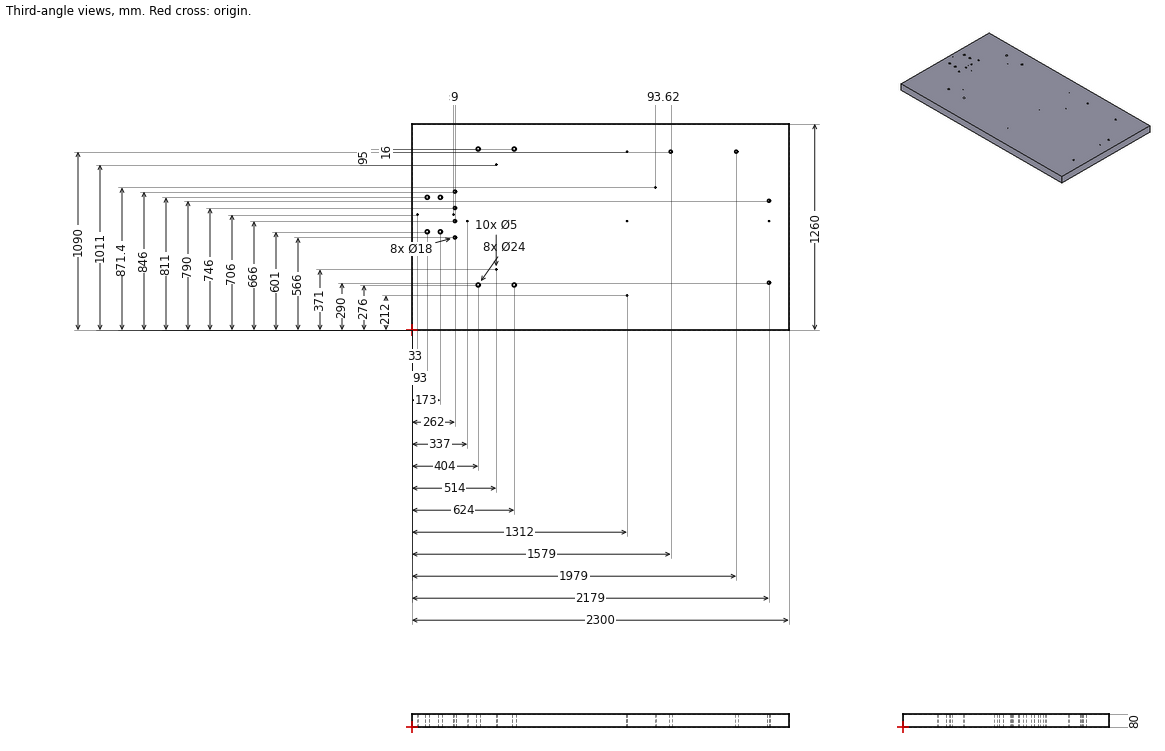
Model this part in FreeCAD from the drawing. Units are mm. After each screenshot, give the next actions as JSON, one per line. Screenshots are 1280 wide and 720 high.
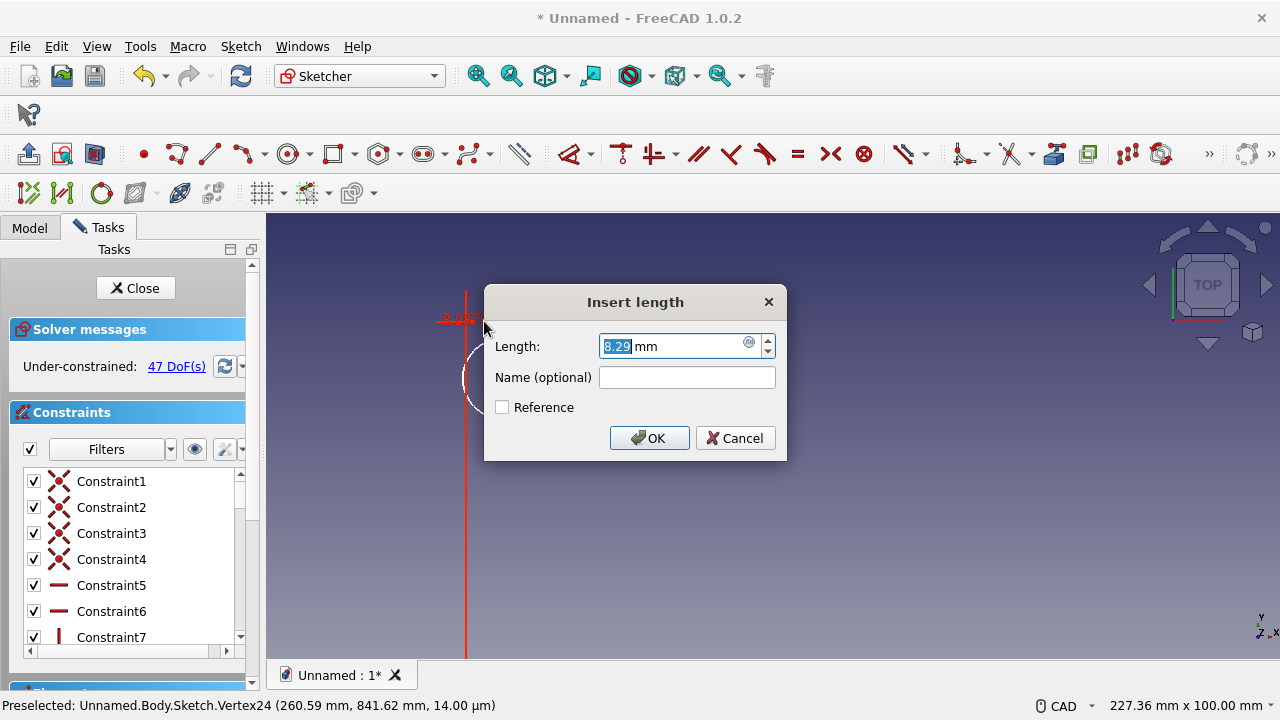
{"action": "type", "text": "9"}
{"action": "key", "text": "Return"}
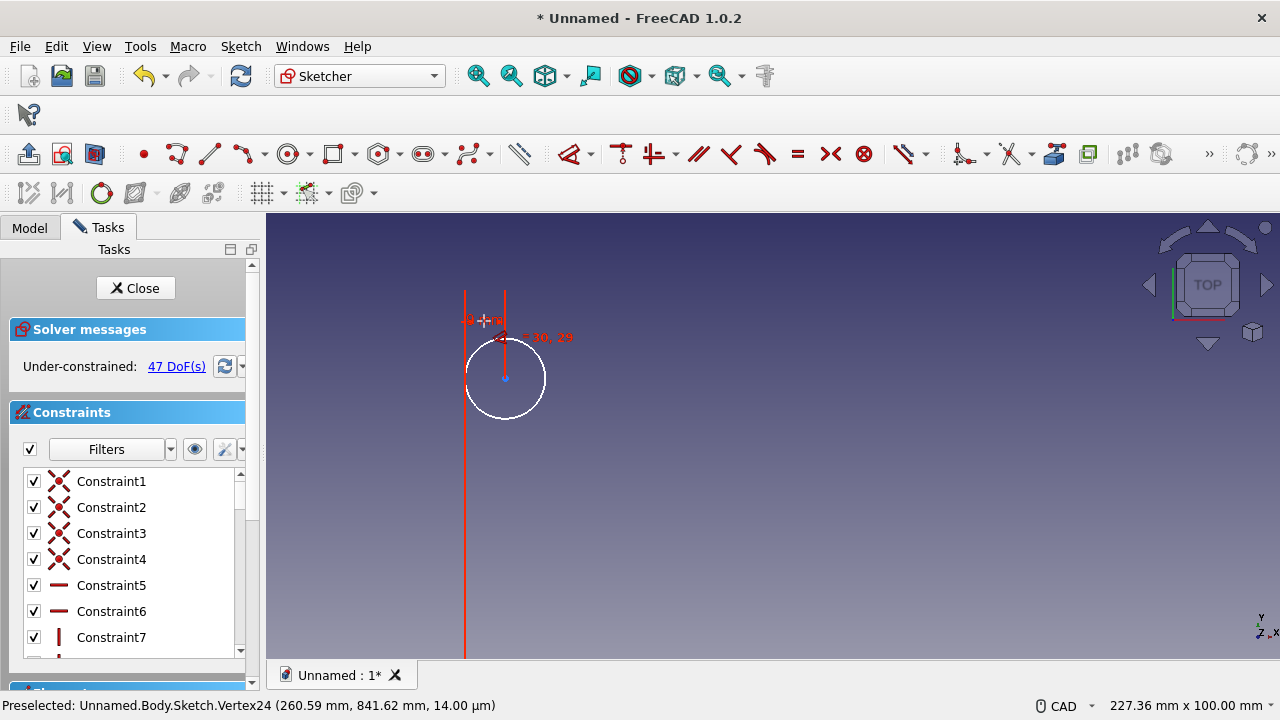
{"action": "scroll", "coordinate": [507, 390], "scroll_direction": "down", "scroll_amount": 15}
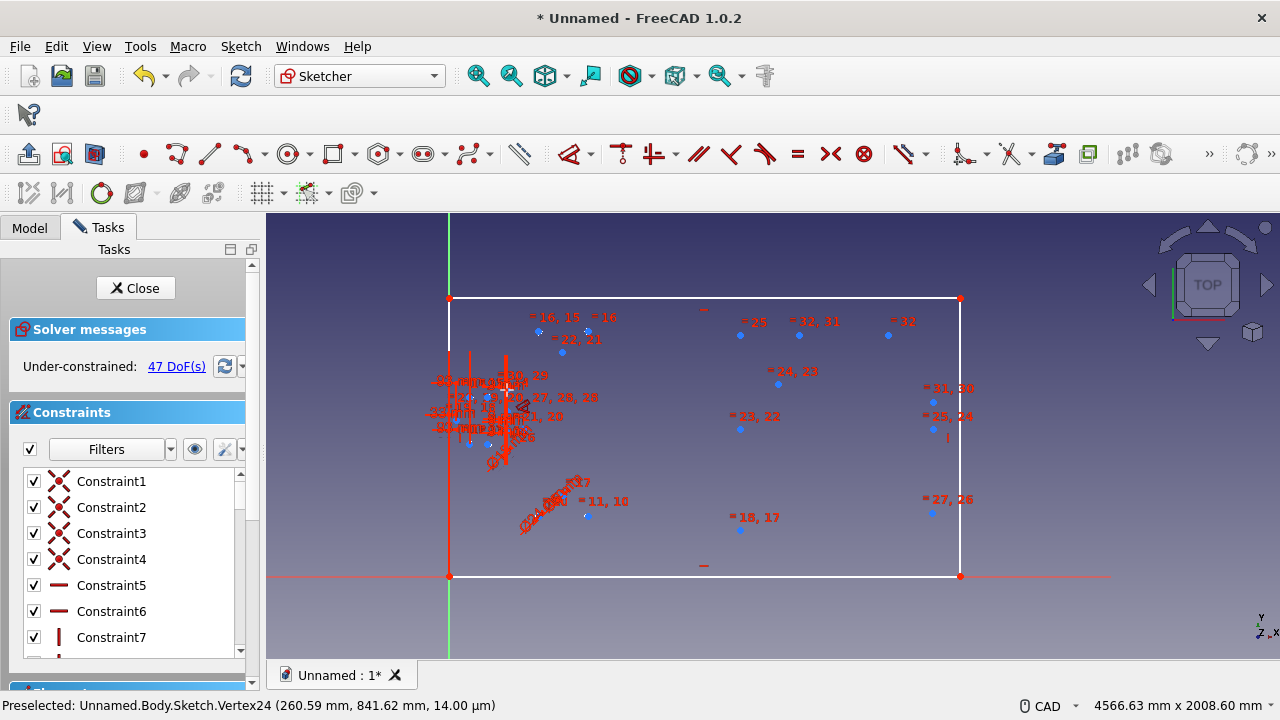
{"action": "left_click", "coordinate": [539, 516]}
{"action": "left_click", "coordinate": [494, 611]}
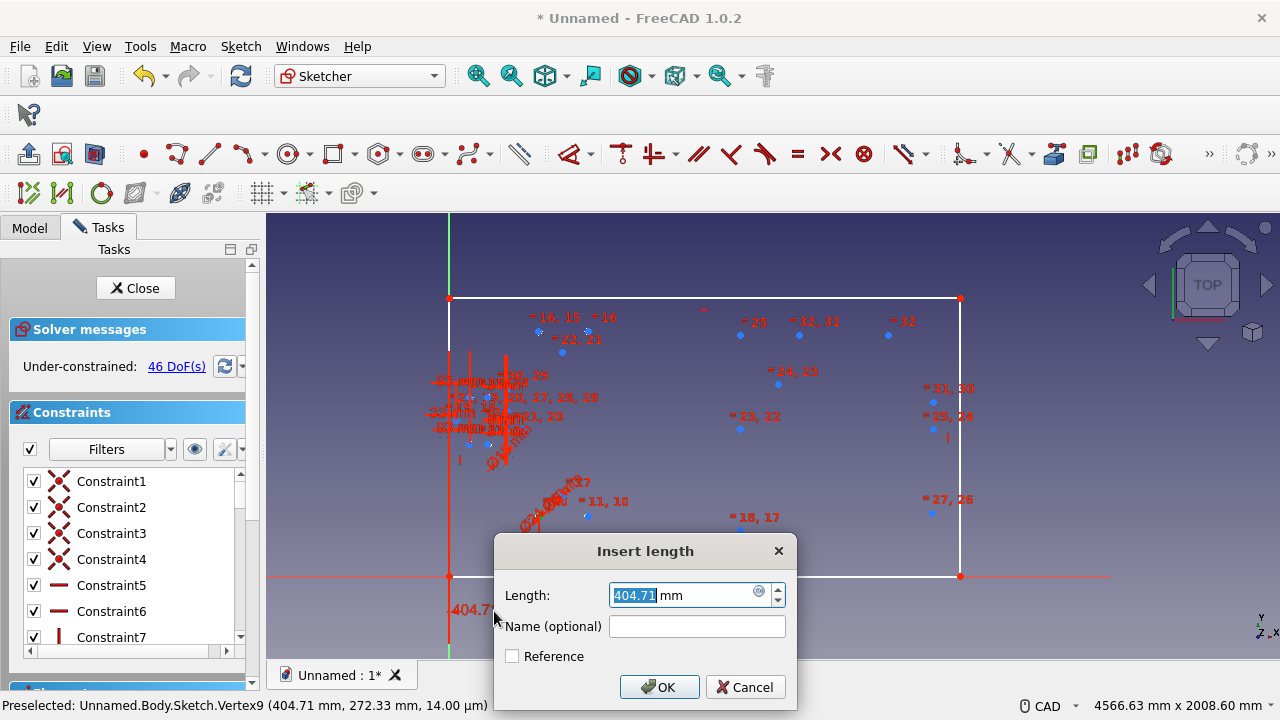
{"action": "type", "text": "404"}
{"action": "key", "text": "Return"}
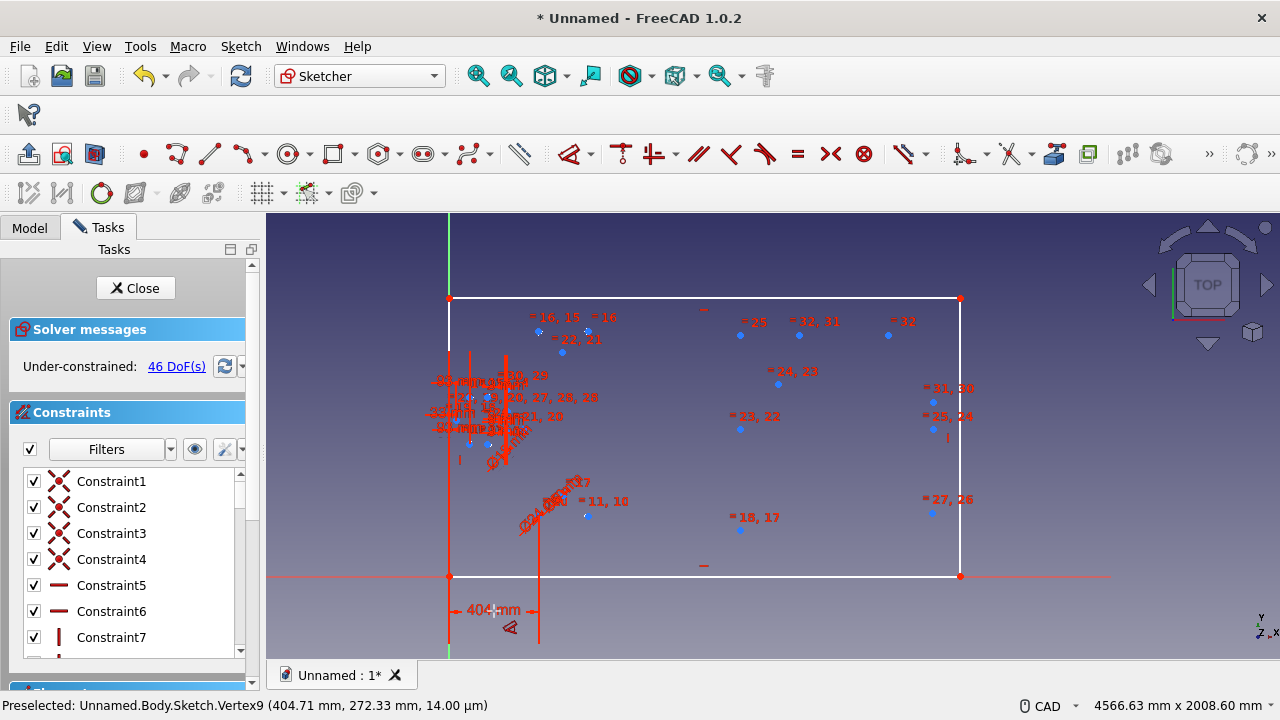
{"action": "left_click", "coordinate": [539, 516]}
{"action": "left_click", "coordinate": [415, 546]}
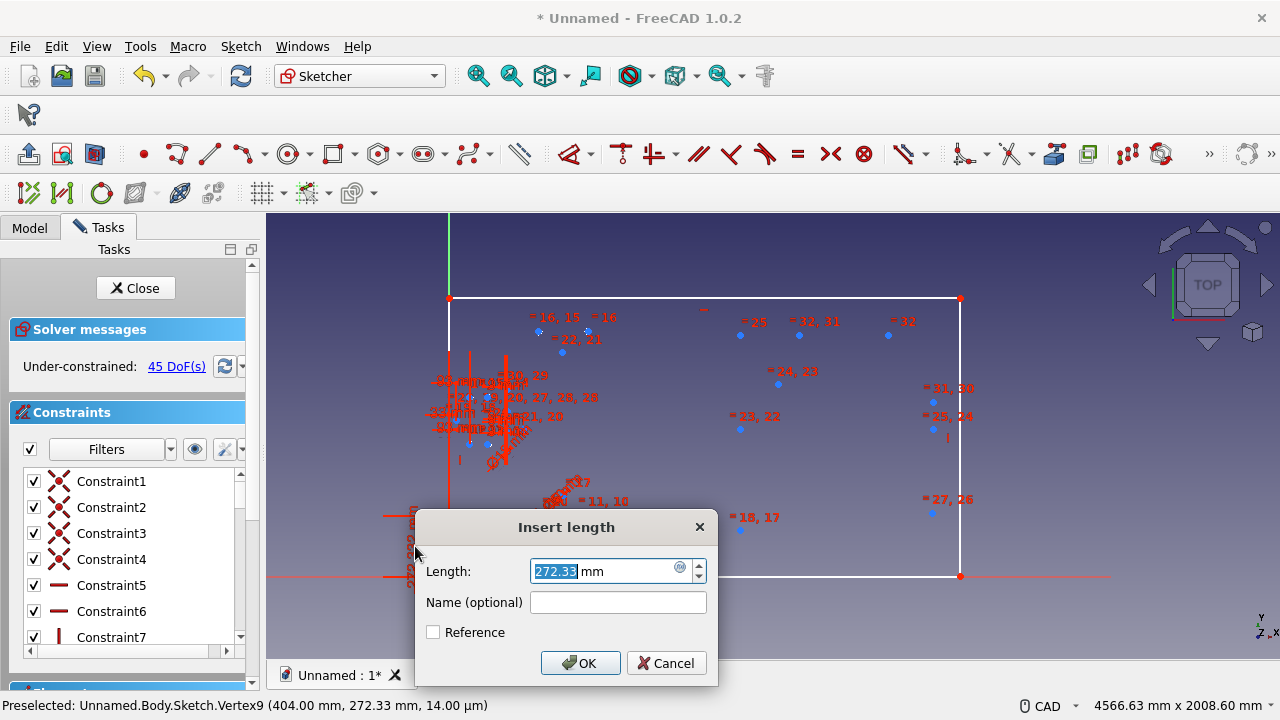
{"action": "type", "text": "276"}
{"action": "key", "text": "Return"}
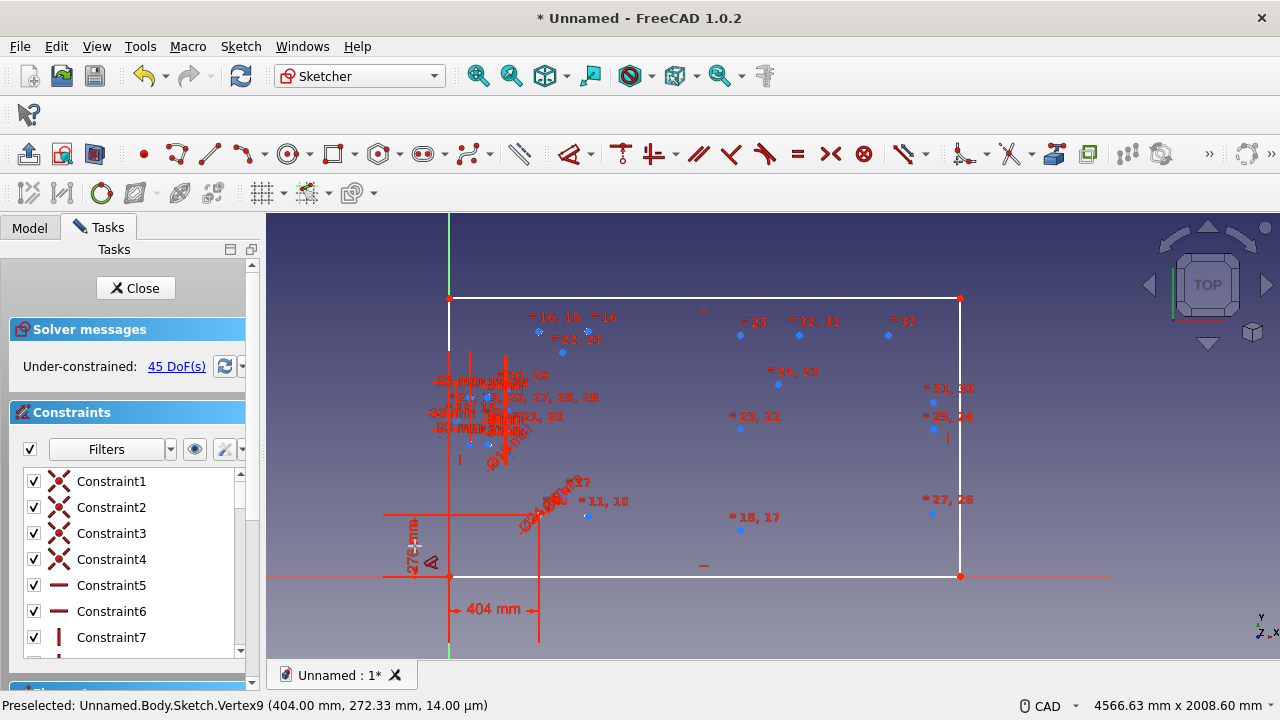
{"action": "left_click", "coordinate": [563, 495]}
{"action": "left_click", "coordinate": [532, 365]}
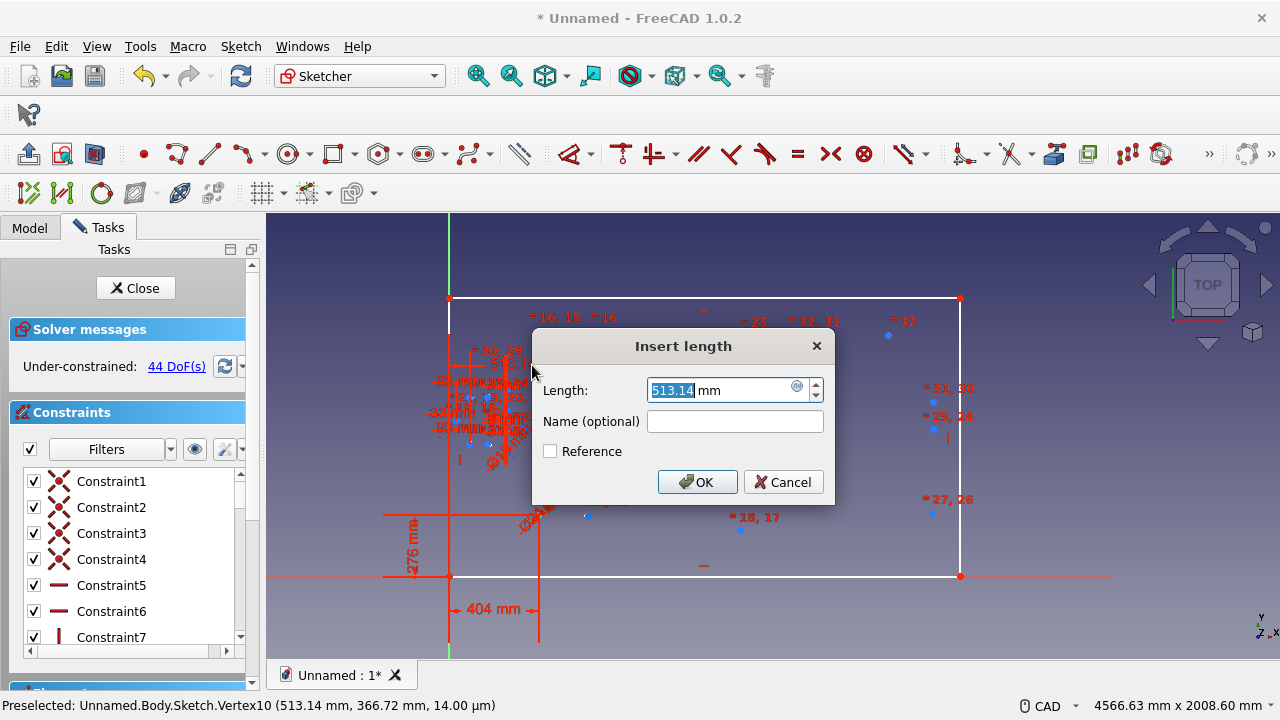
{"action": "type", "text": "514"}
{"action": "key", "text": "Return"}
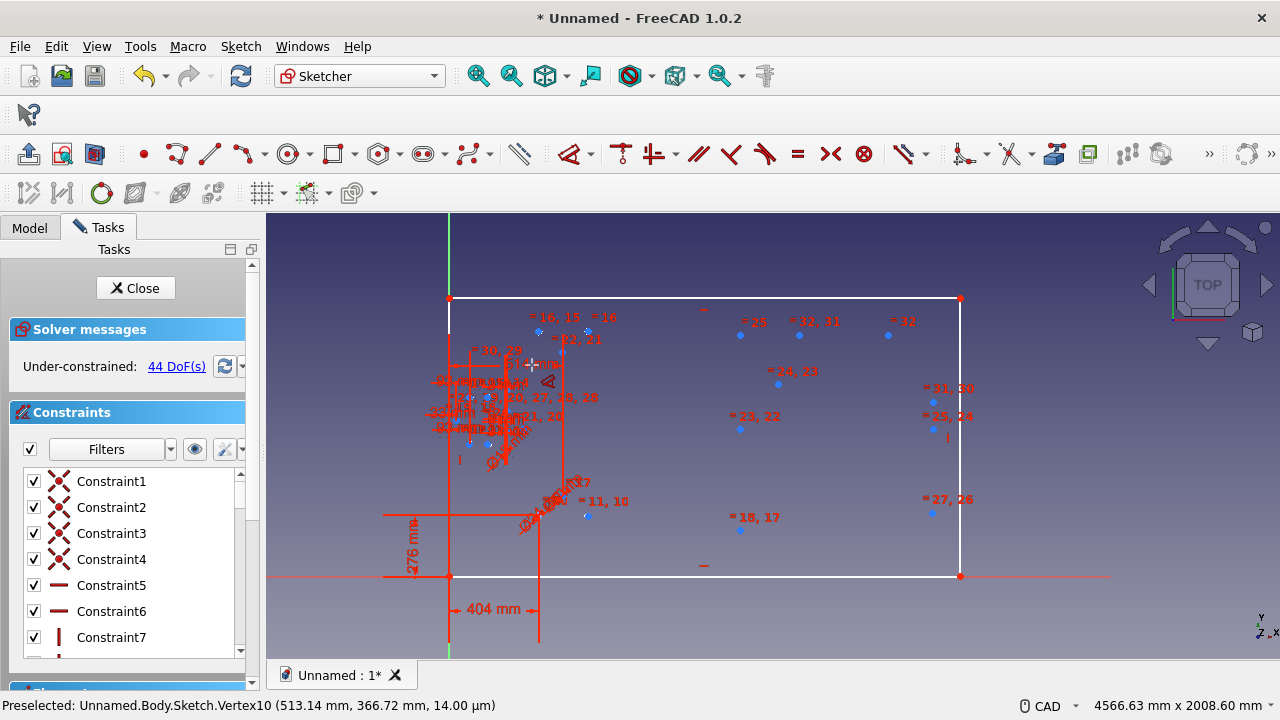
{"action": "left_click", "coordinate": [563, 495]}
{"action": "left_click", "coordinate": [415, 517]}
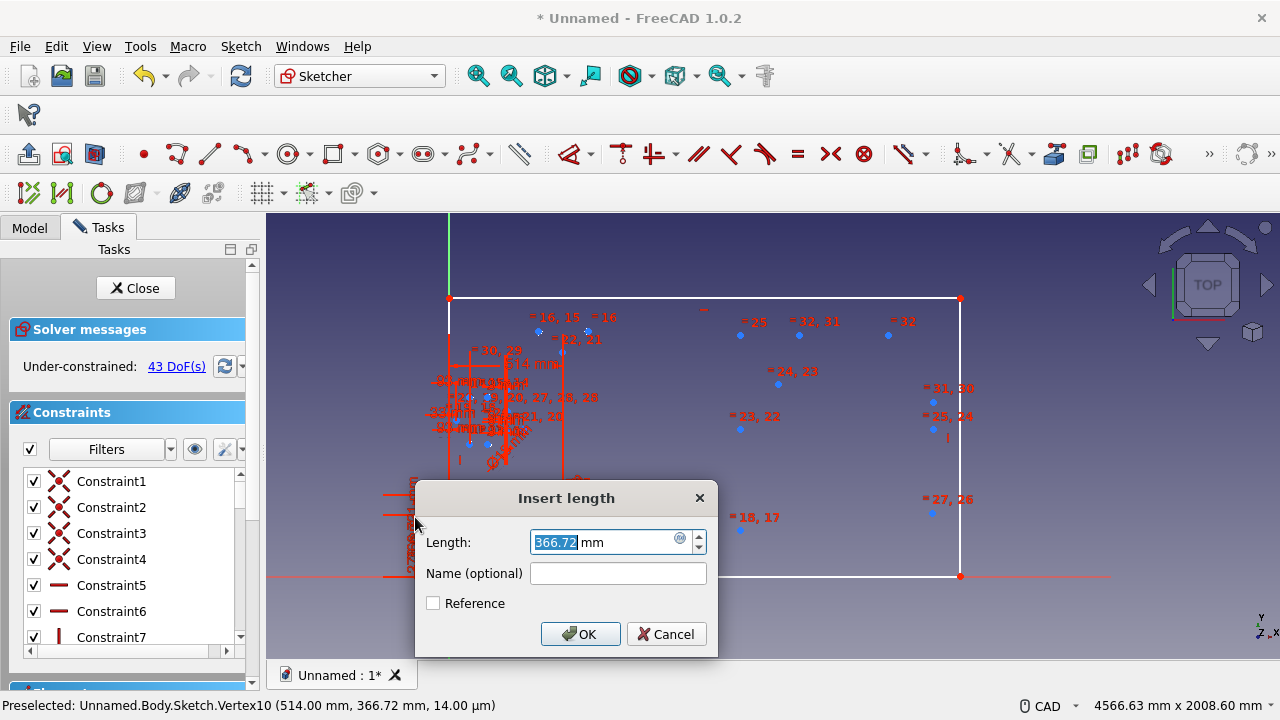
{"action": "type", "text": "371"}
{"action": "key", "text": "Return"}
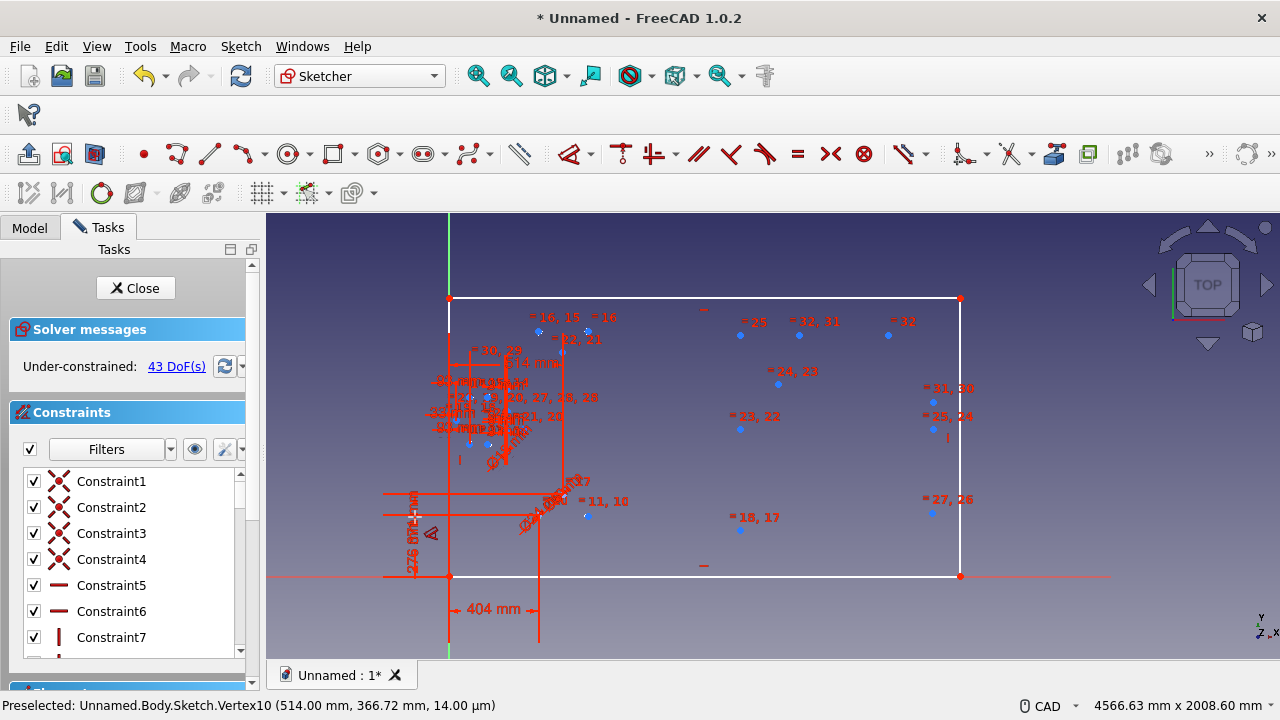
{"action": "left_click", "coordinate": [588, 516]}
{"action": "left_click", "coordinate": [567, 611]}